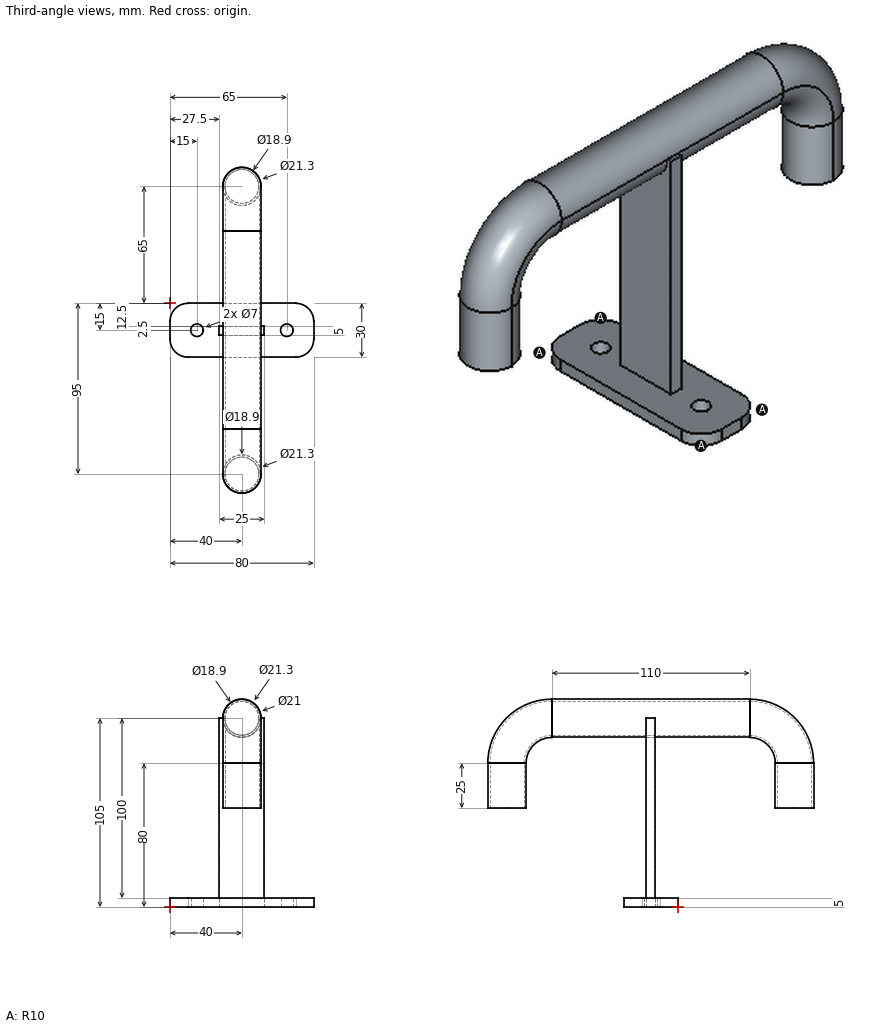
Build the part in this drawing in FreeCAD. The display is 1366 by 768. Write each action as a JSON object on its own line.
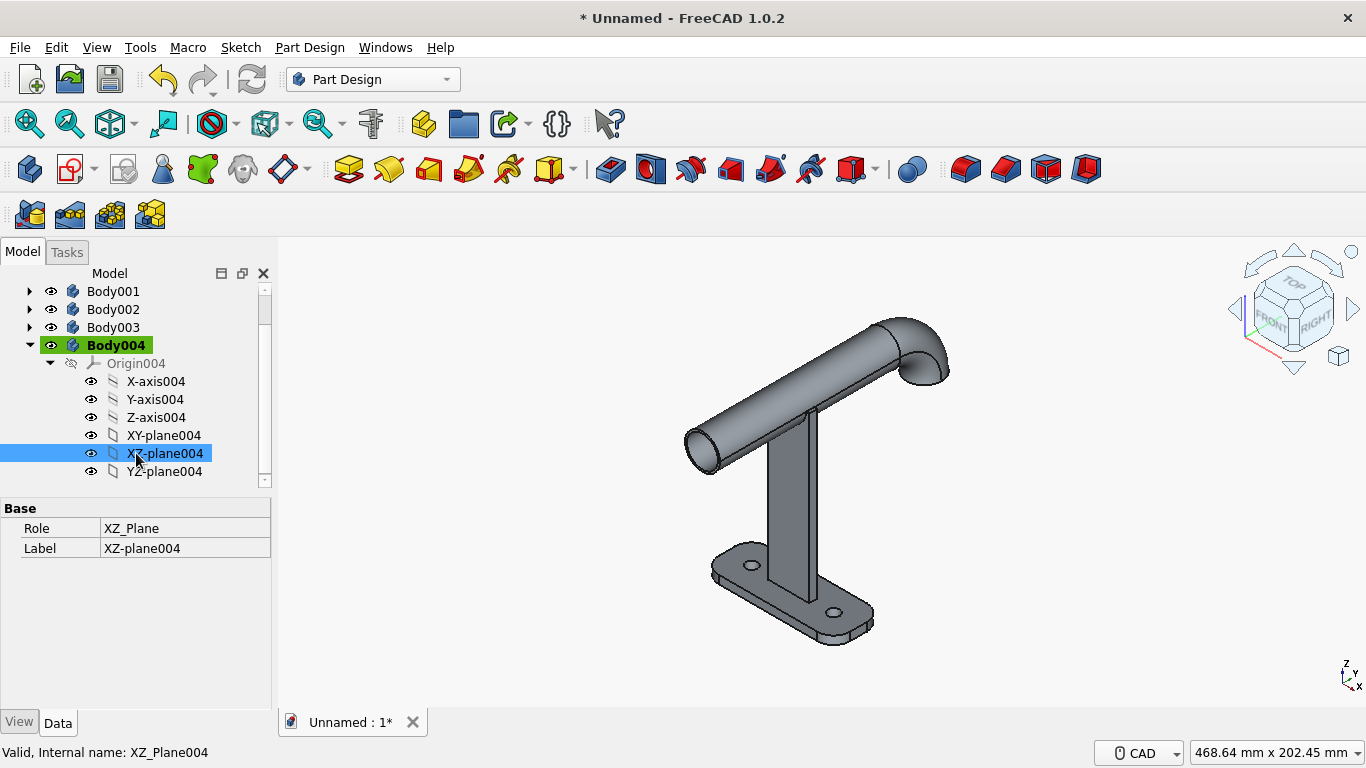
{"action": "left_click", "coordinate": [284, 170]}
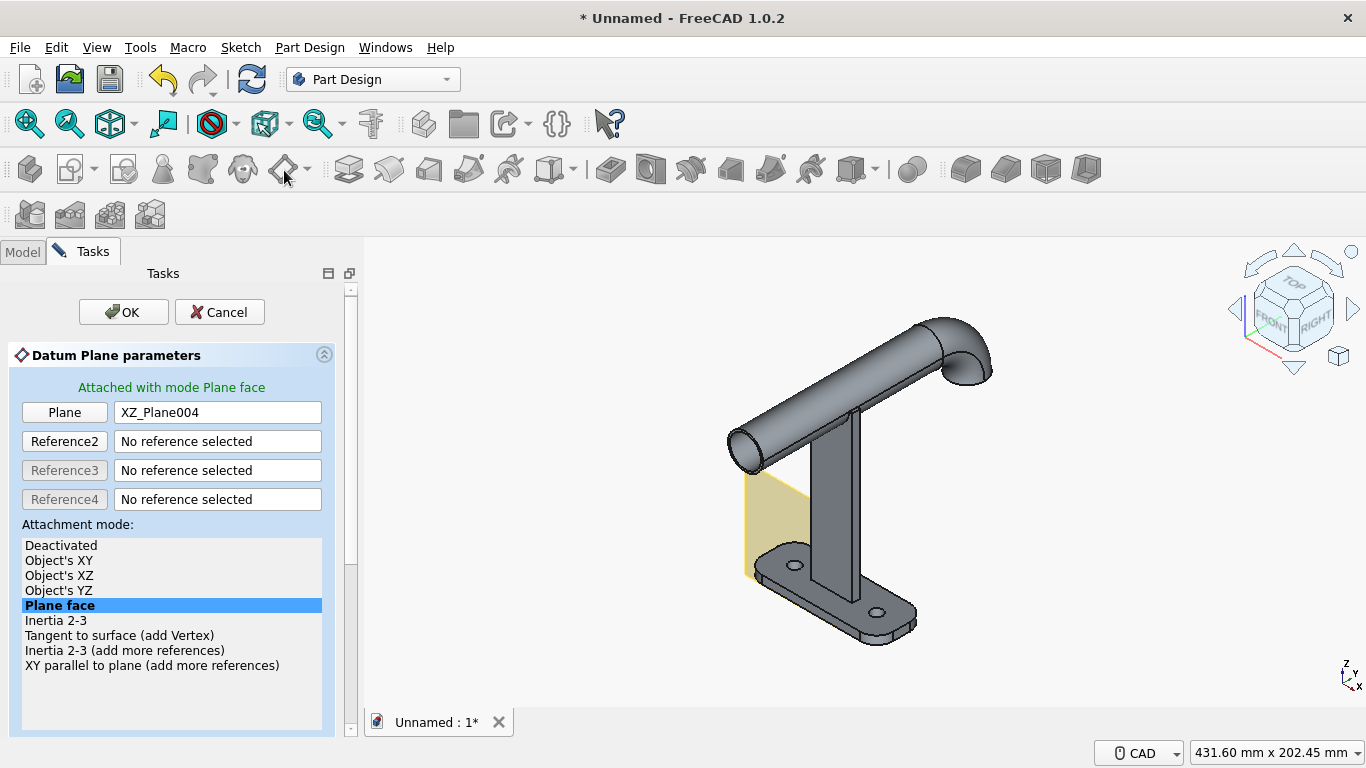
{"action": "scroll", "coordinate": [351, 510], "scroll_direction": "down", "scroll_amount": 3}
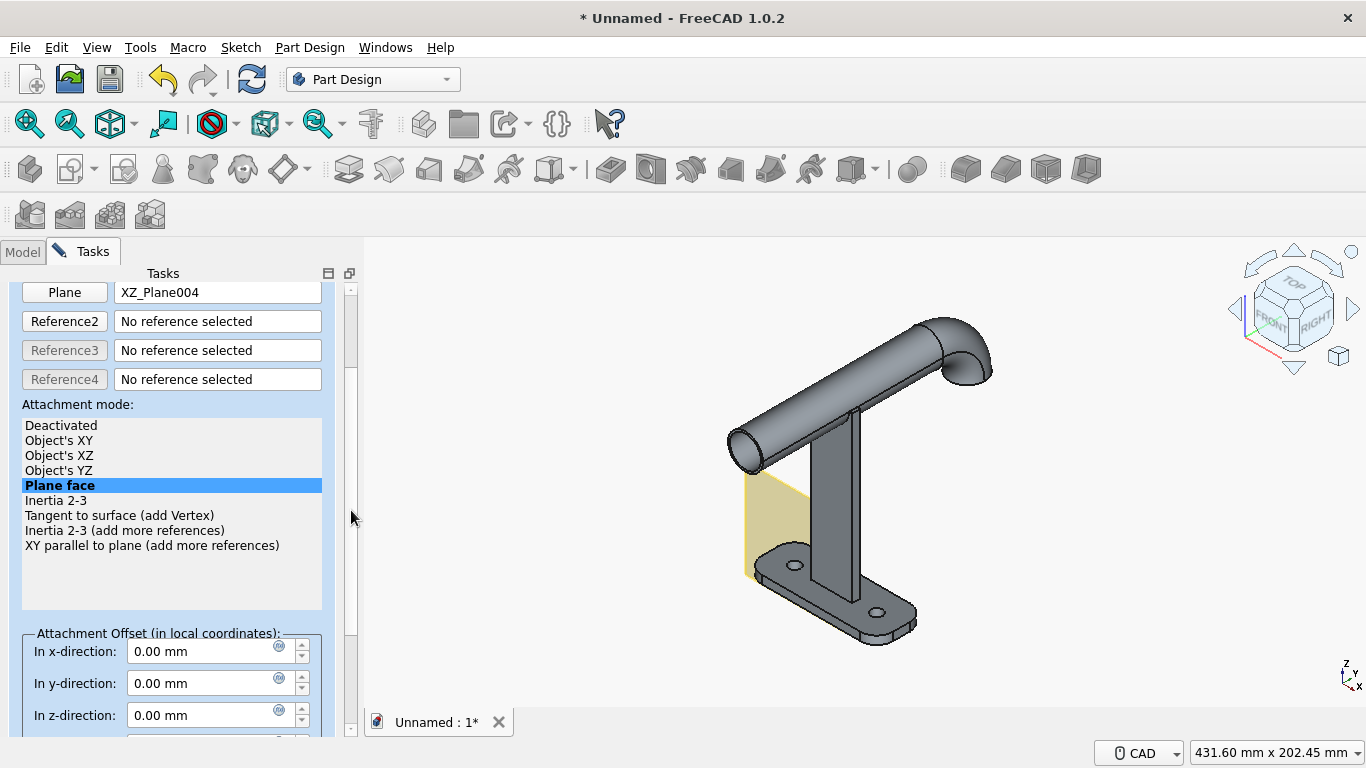
{"action": "triple_click", "coordinate": [210, 655]}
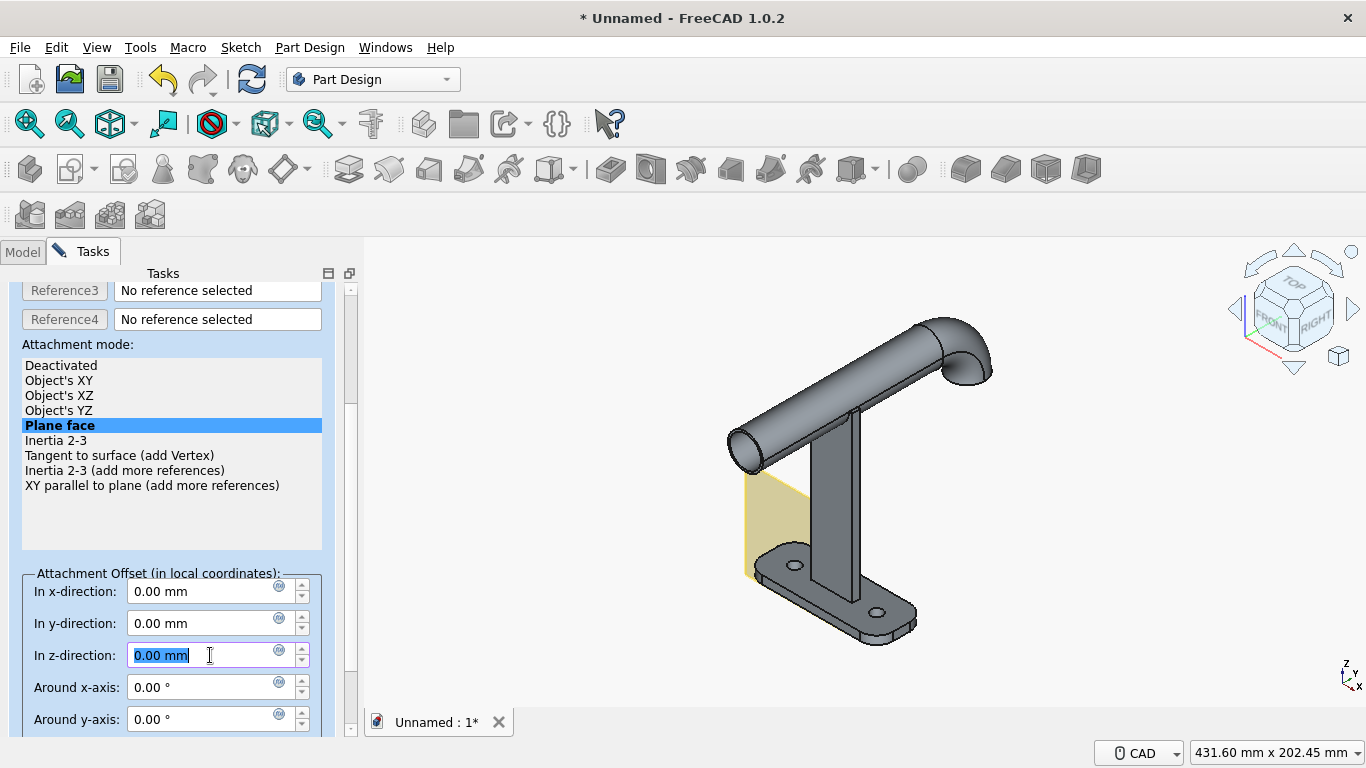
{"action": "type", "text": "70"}
{"action": "key", "text": "Tab"}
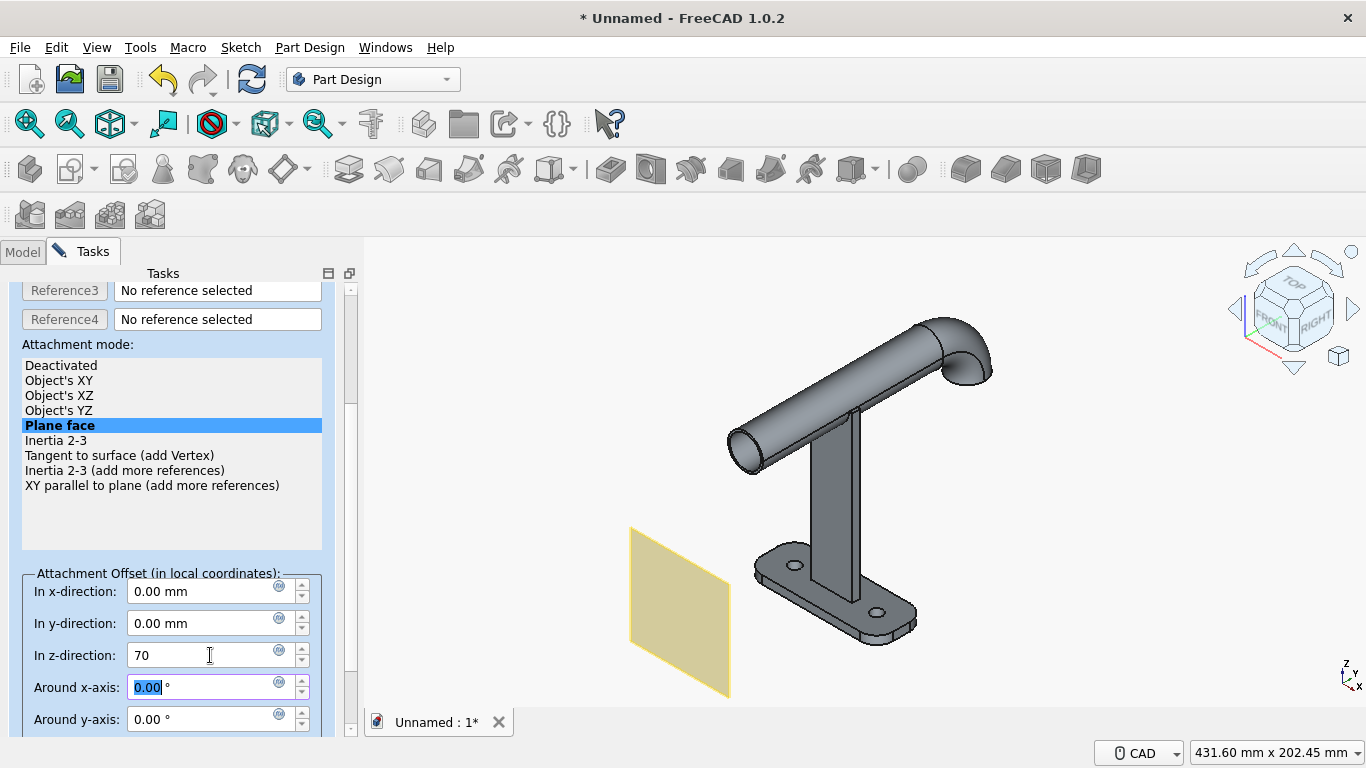
{"action": "scroll", "coordinate": [351, 510], "scroll_direction": "up", "scroll_amount": 4}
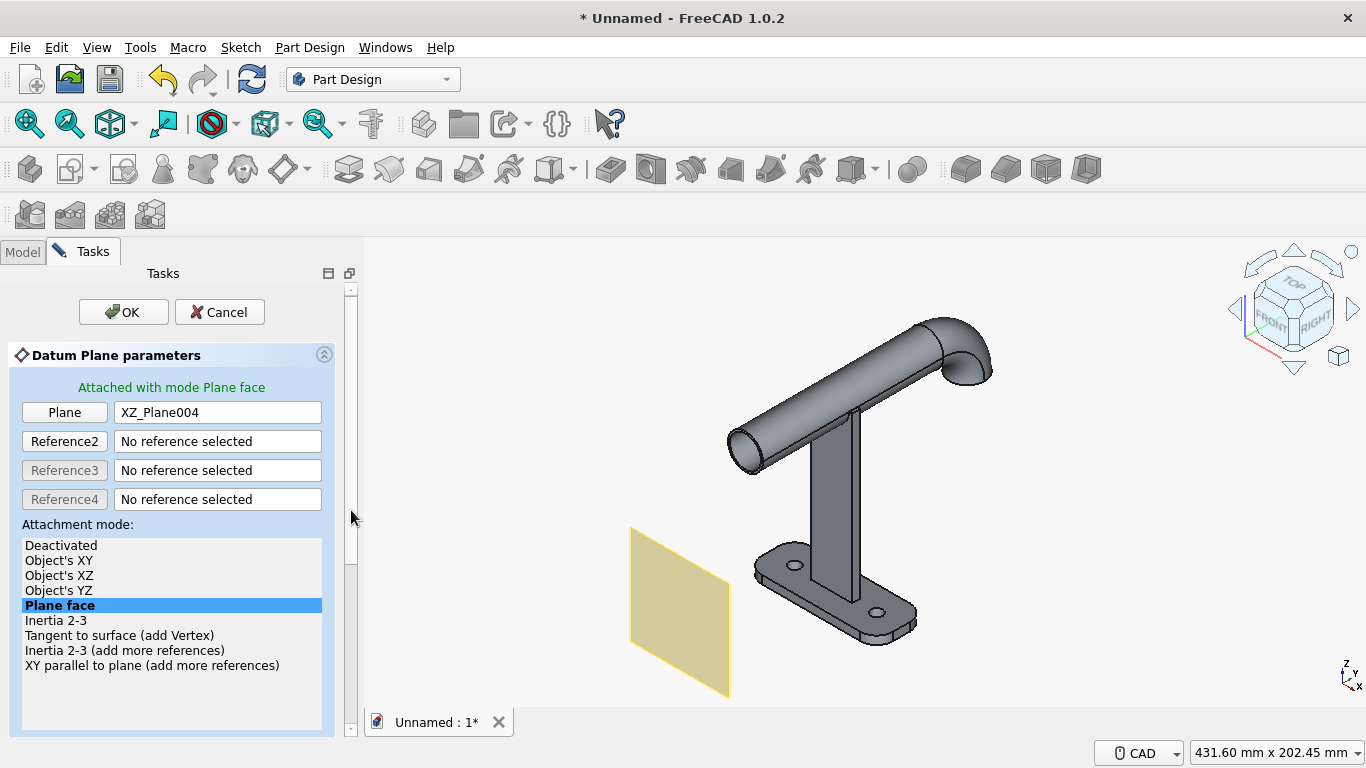
{"action": "left_click", "coordinate": [124, 312]}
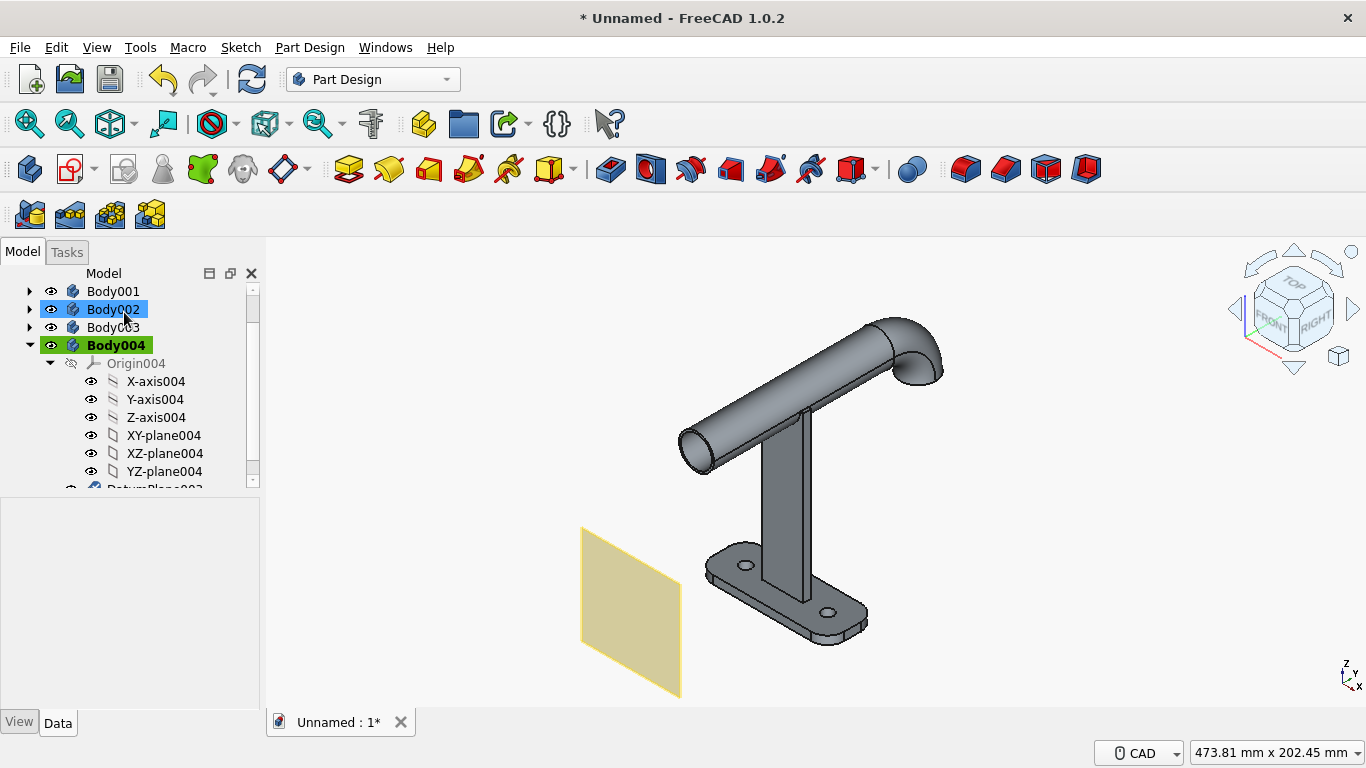
{"action": "scroll", "coordinate": [120, 377], "scroll_direction": "down", "scroll_amount": 3}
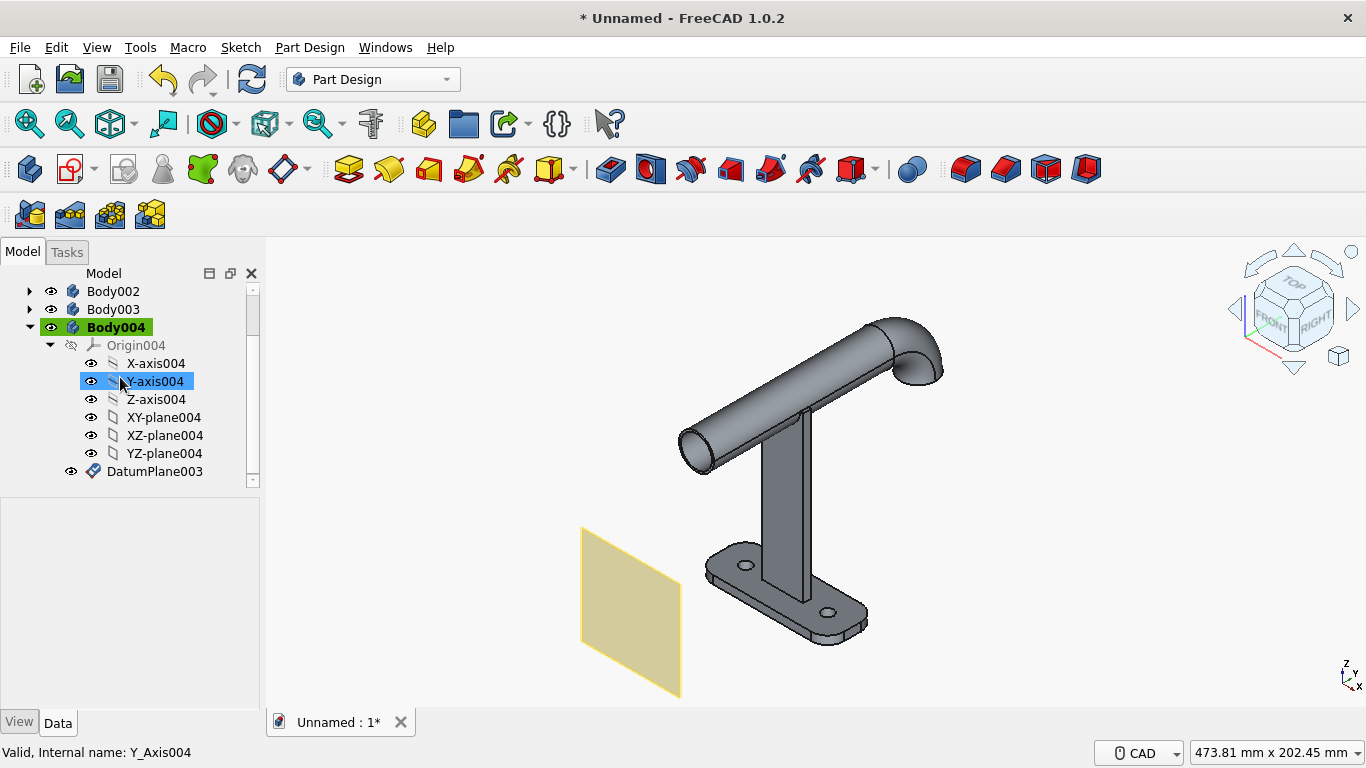
{"action": "left_click", "coordinate": [116, 471]}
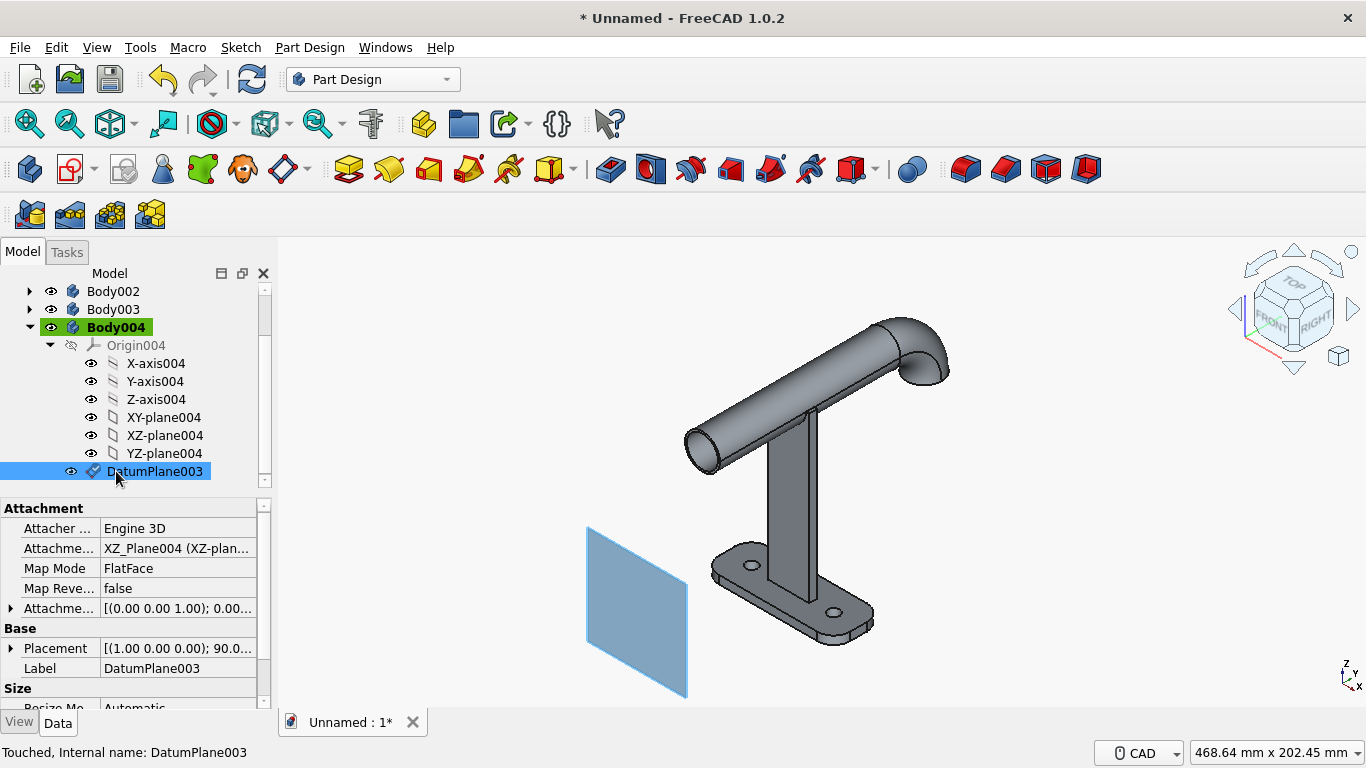
{"action": "left_click", "coordinate": [70, 170]}